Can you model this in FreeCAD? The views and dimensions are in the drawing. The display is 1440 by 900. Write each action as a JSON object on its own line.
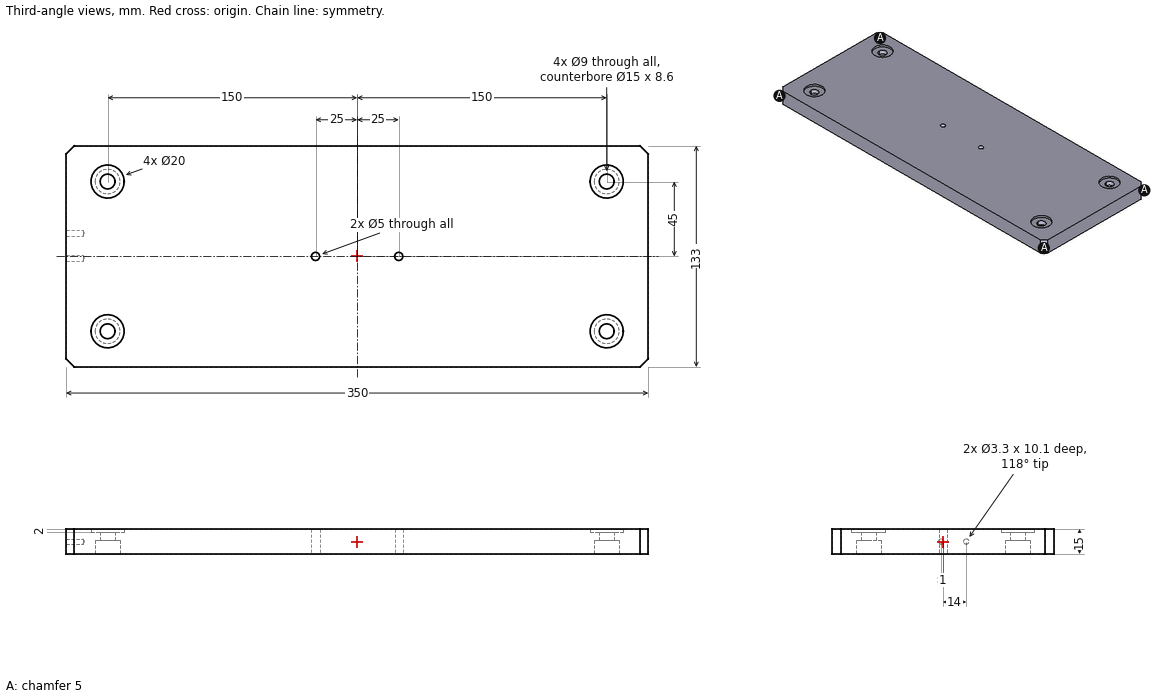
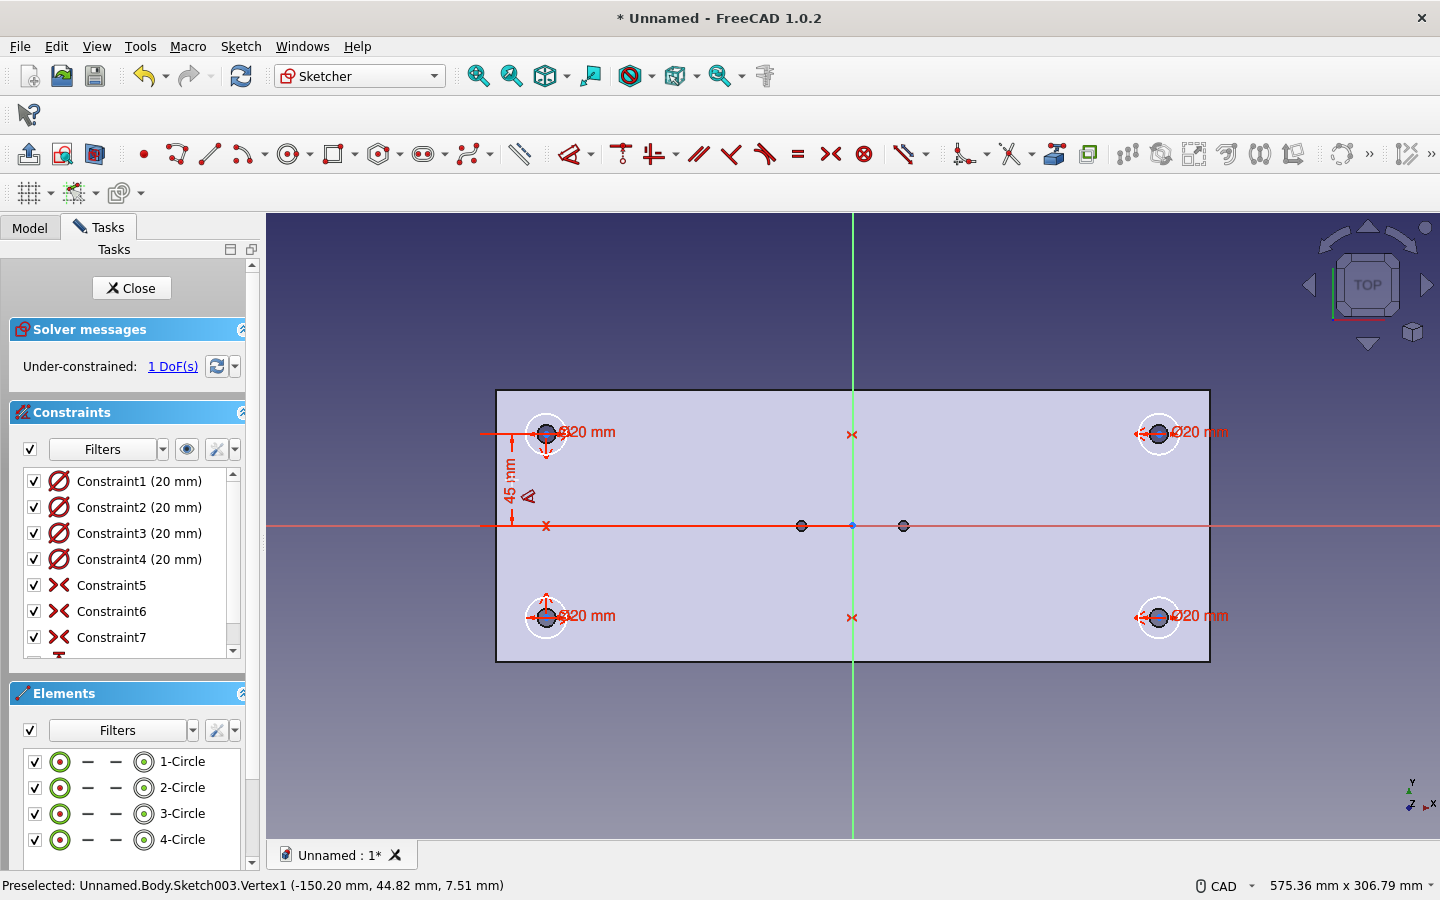
{"action": "left_click", "coordinate": [546, 434]}
{"action": "left_click", "coordinate": [699, 400]}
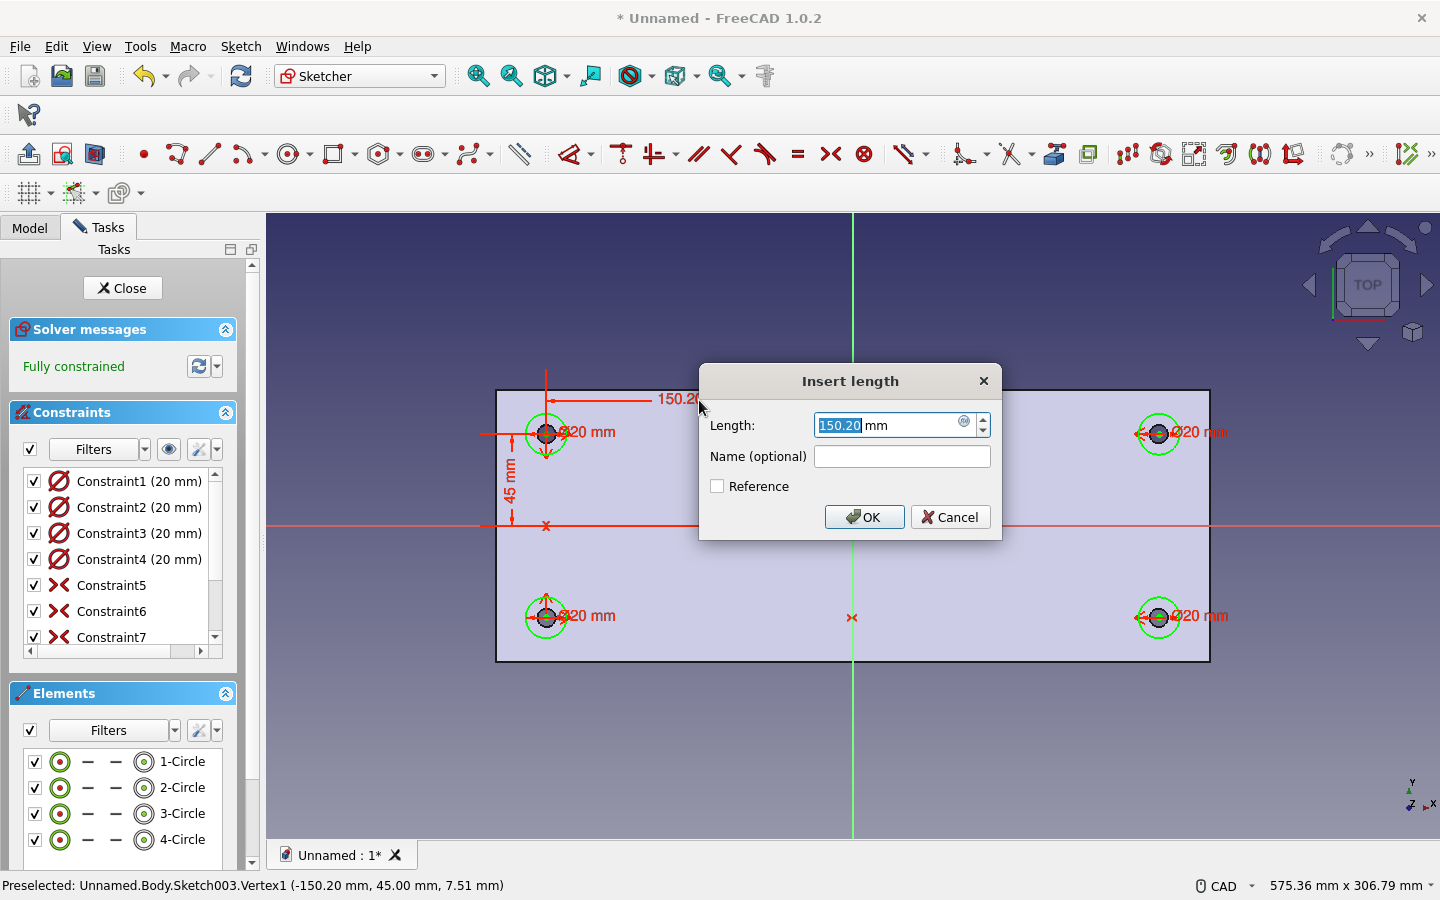
{"action": "type", "text": "150"}
{"action": "key", "text": "Return"}
{"action": "key", "text": "Escape"}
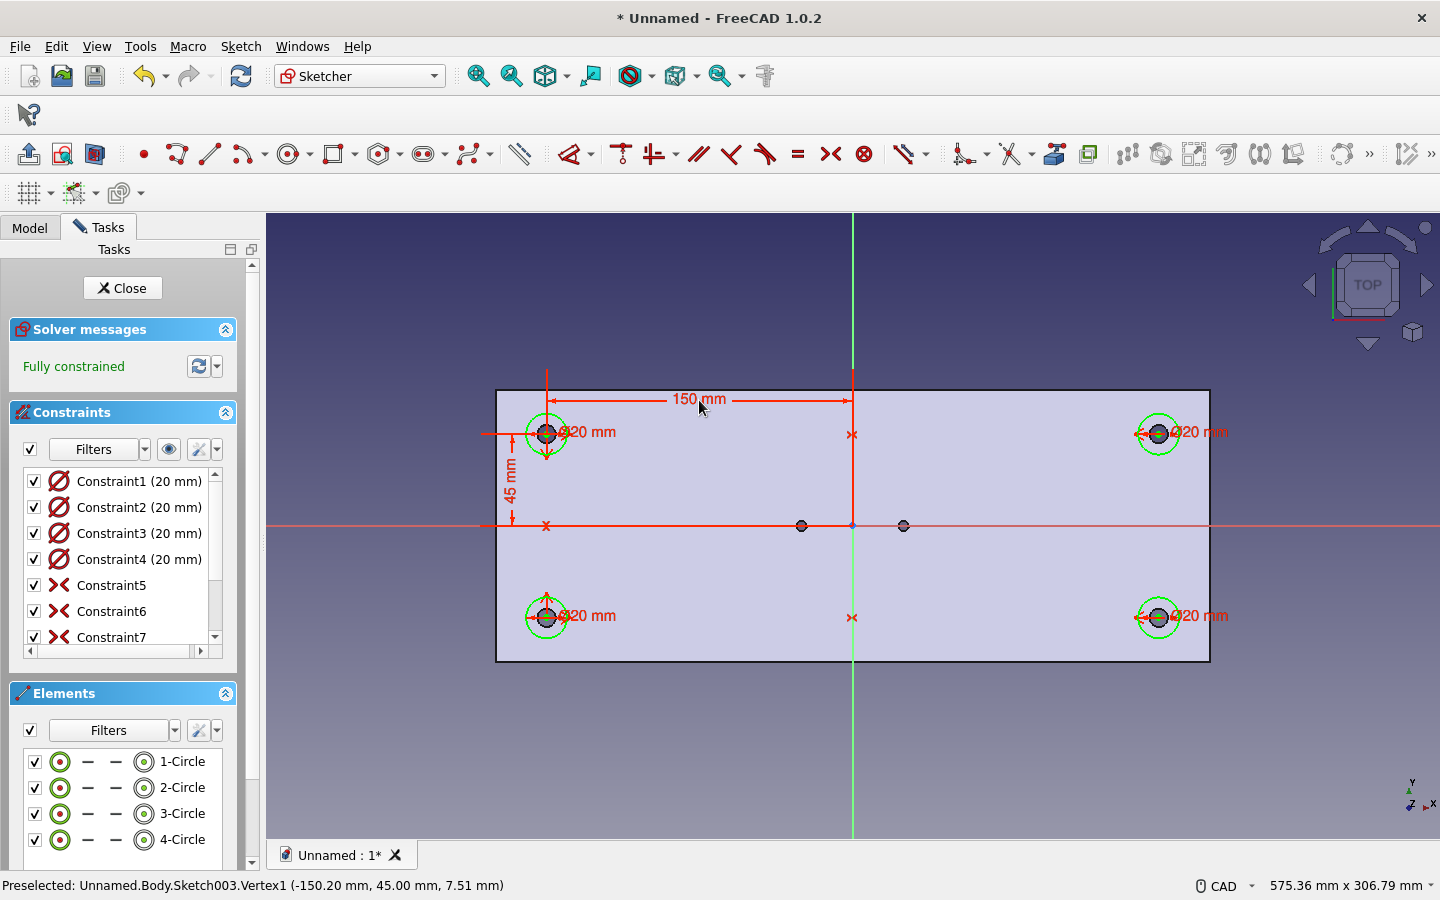
{"action": "left_click", "coordinate": [123, 288]}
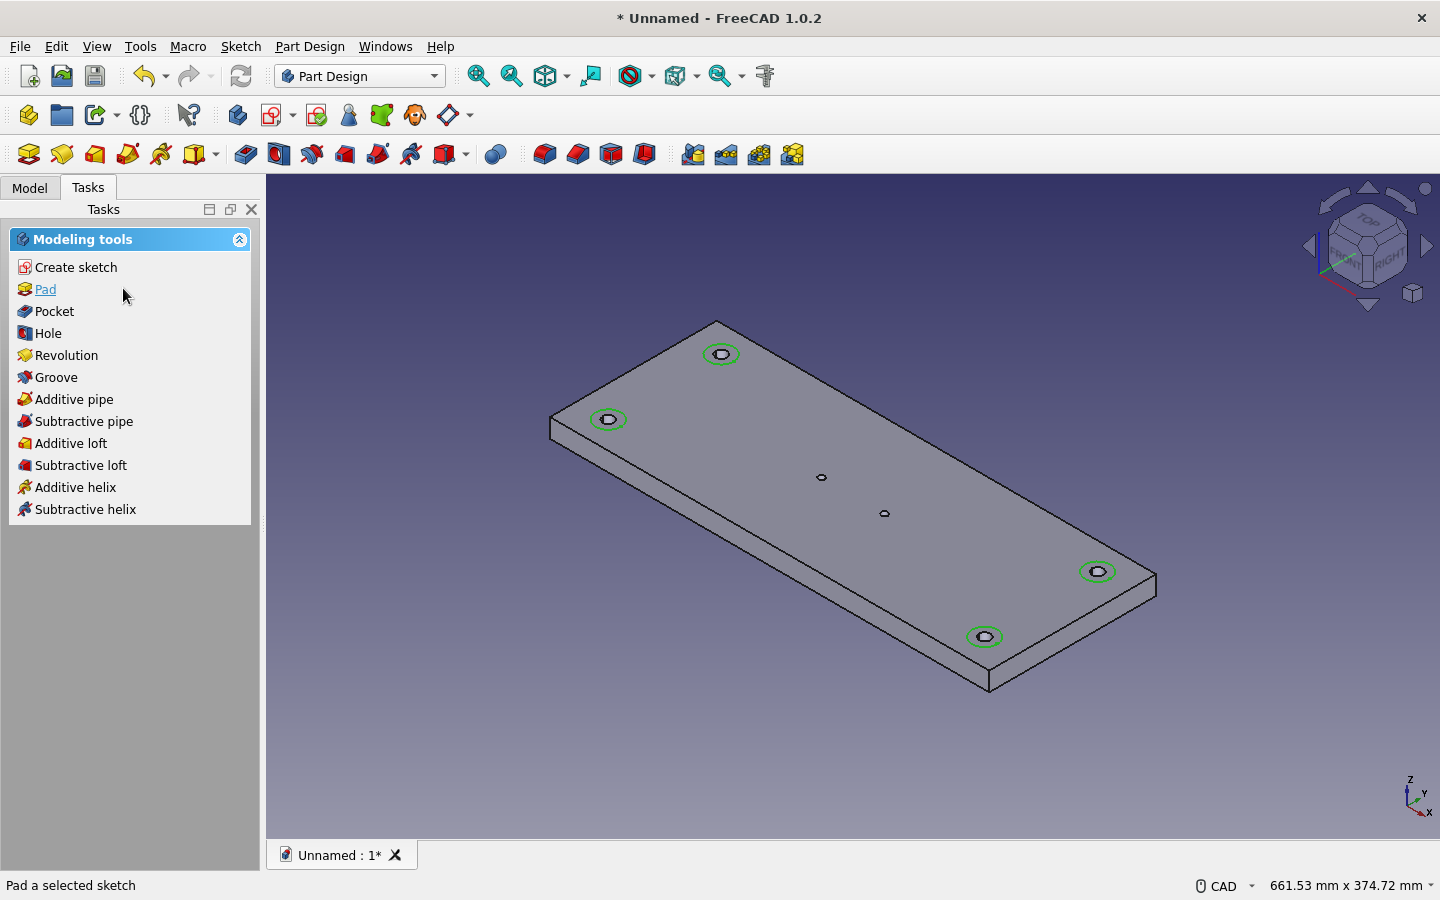
{"action": "left_click", "coordinate": [246, 154]}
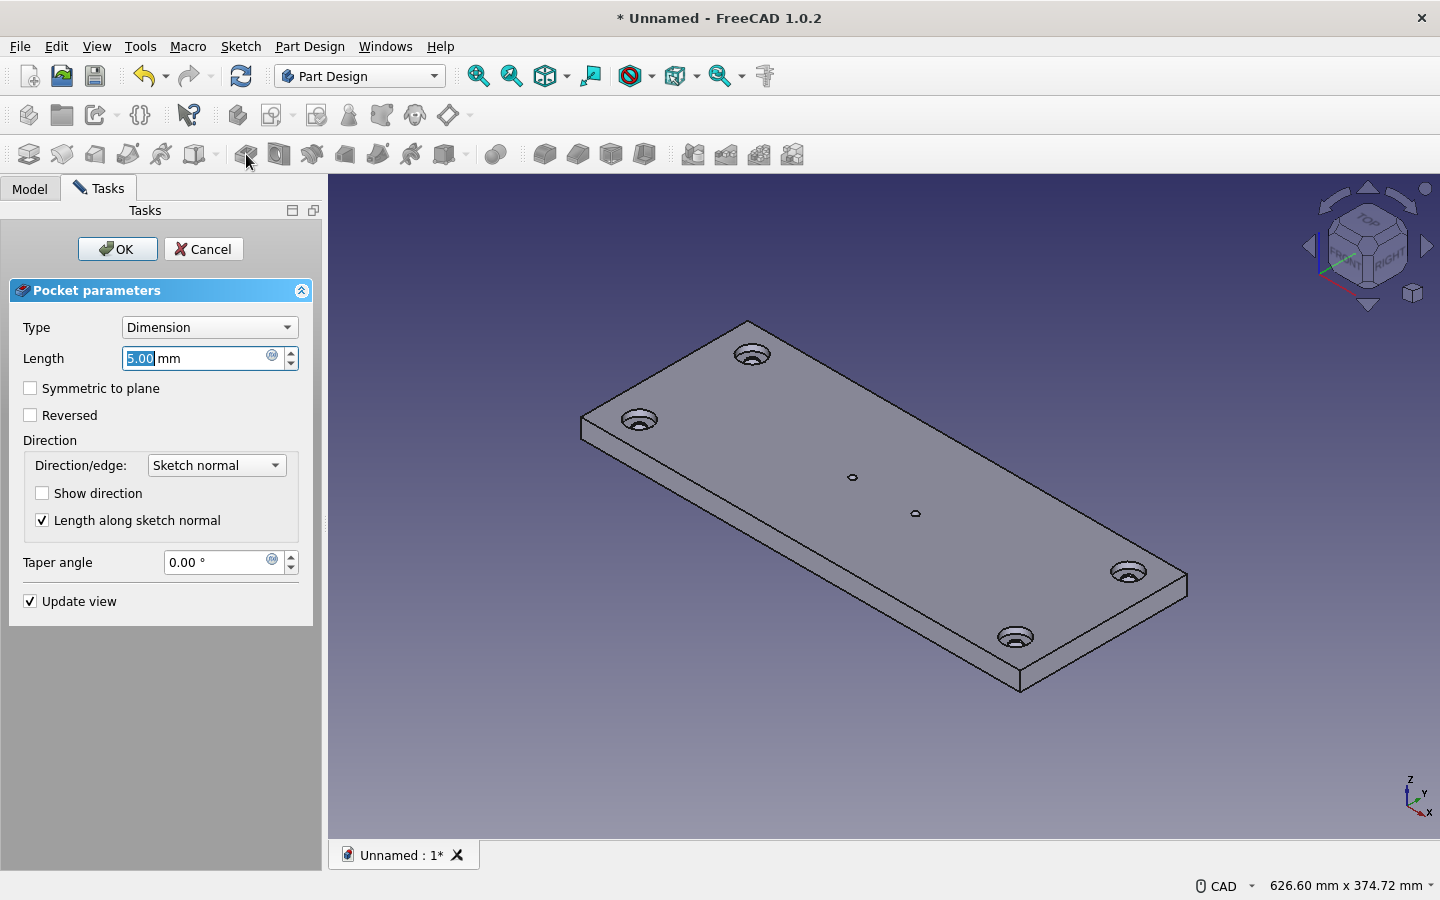
{"action": "type", "text": "2"}
{"action": "key", "text": "Tab"}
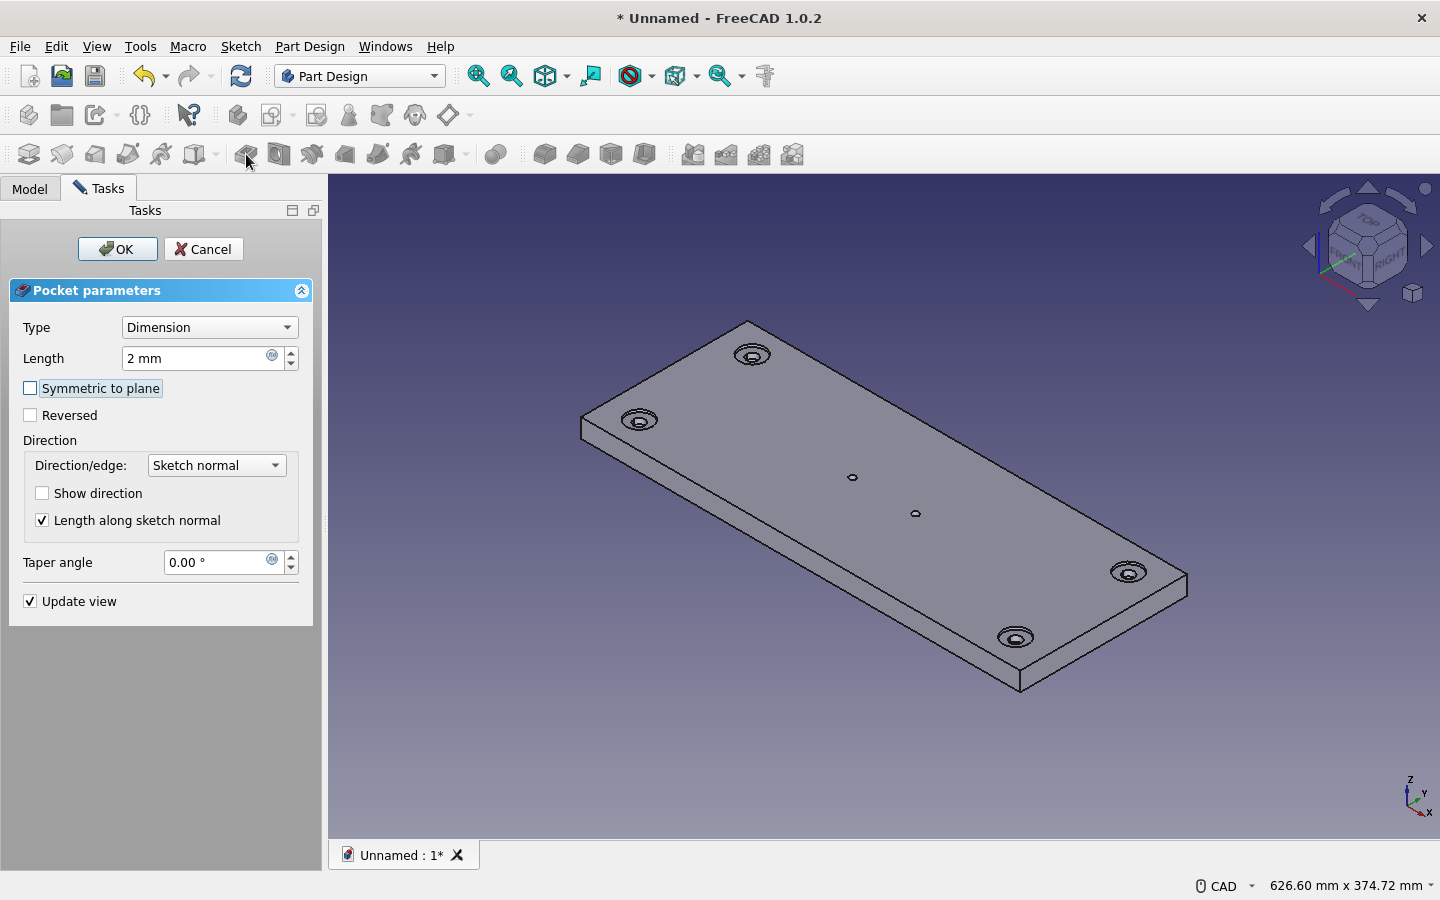
{"action": "left_click", "coordinate": [118, 249]}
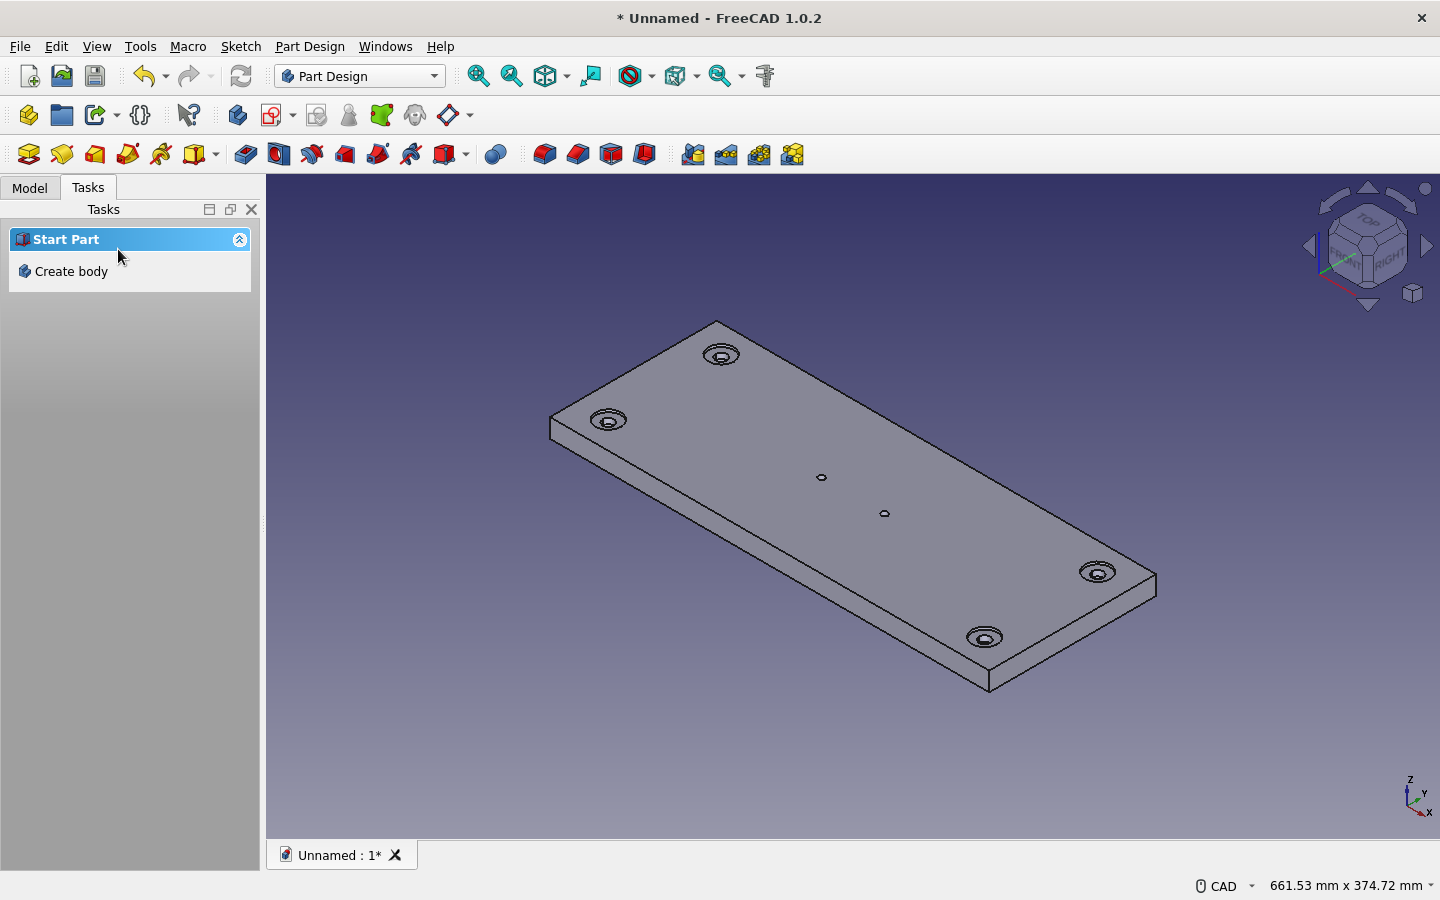
{"action": "key", "text": "6"}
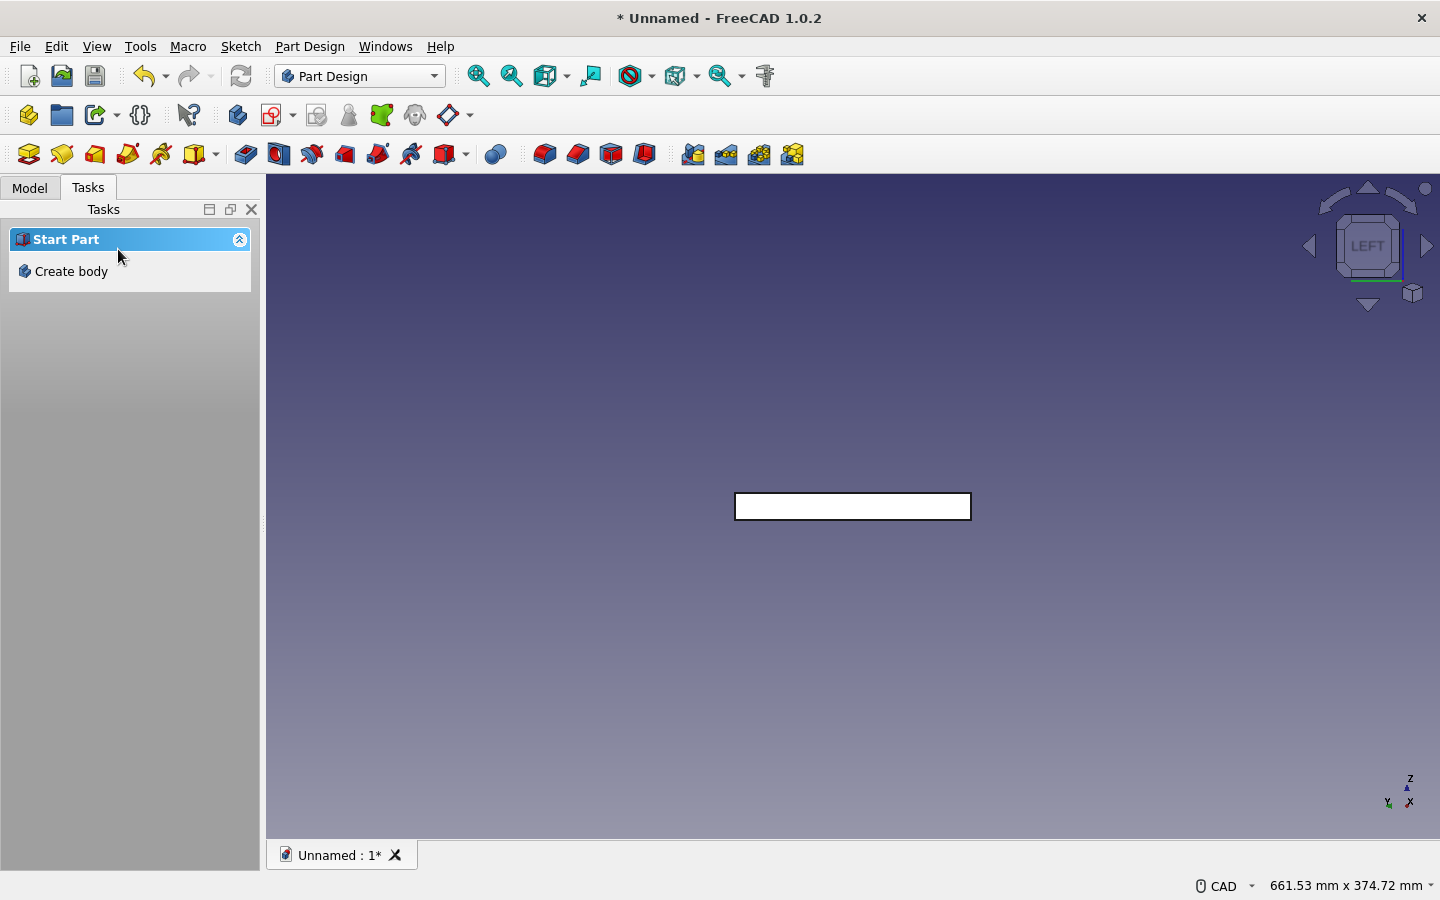
{"action": "key", "text": "v f"}